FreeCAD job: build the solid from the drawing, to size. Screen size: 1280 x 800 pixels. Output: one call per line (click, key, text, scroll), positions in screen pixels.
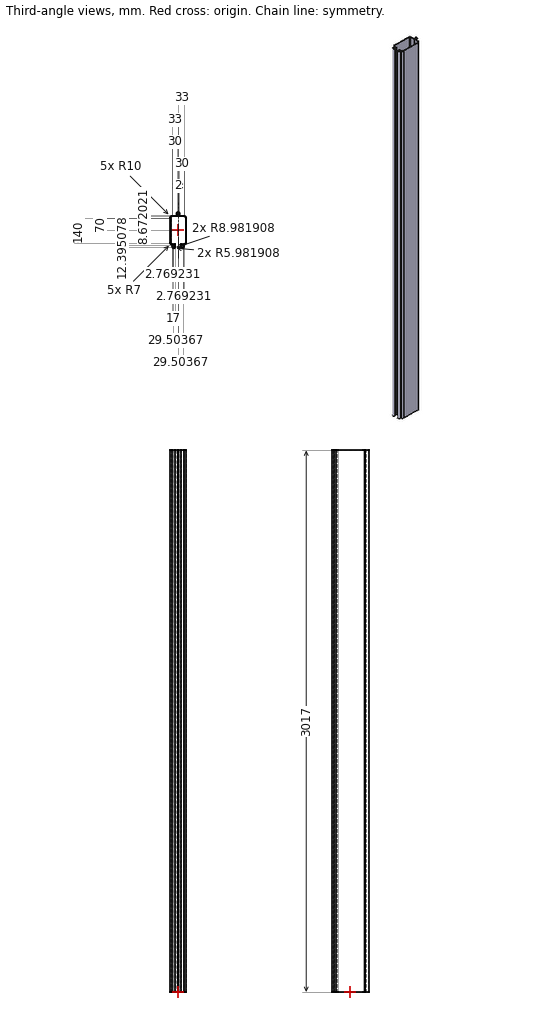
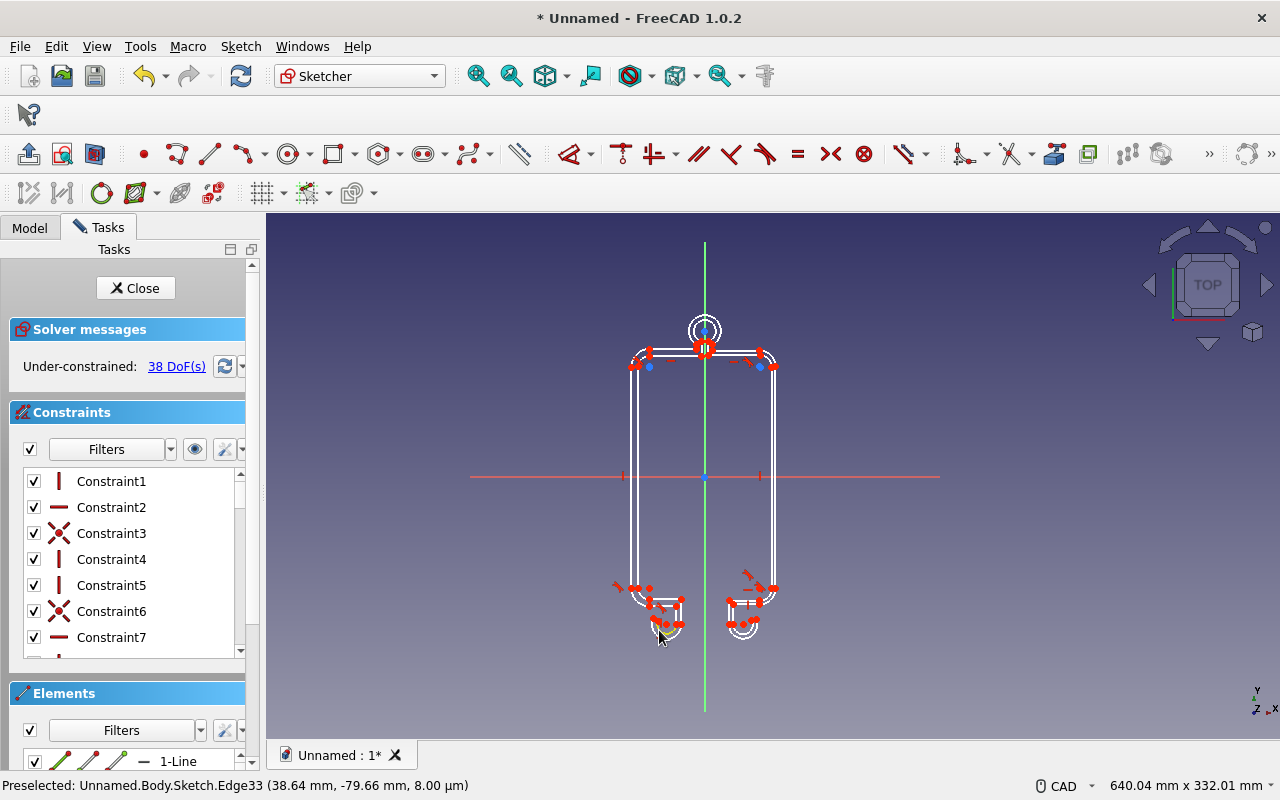
scroll(771, 362, up, 7)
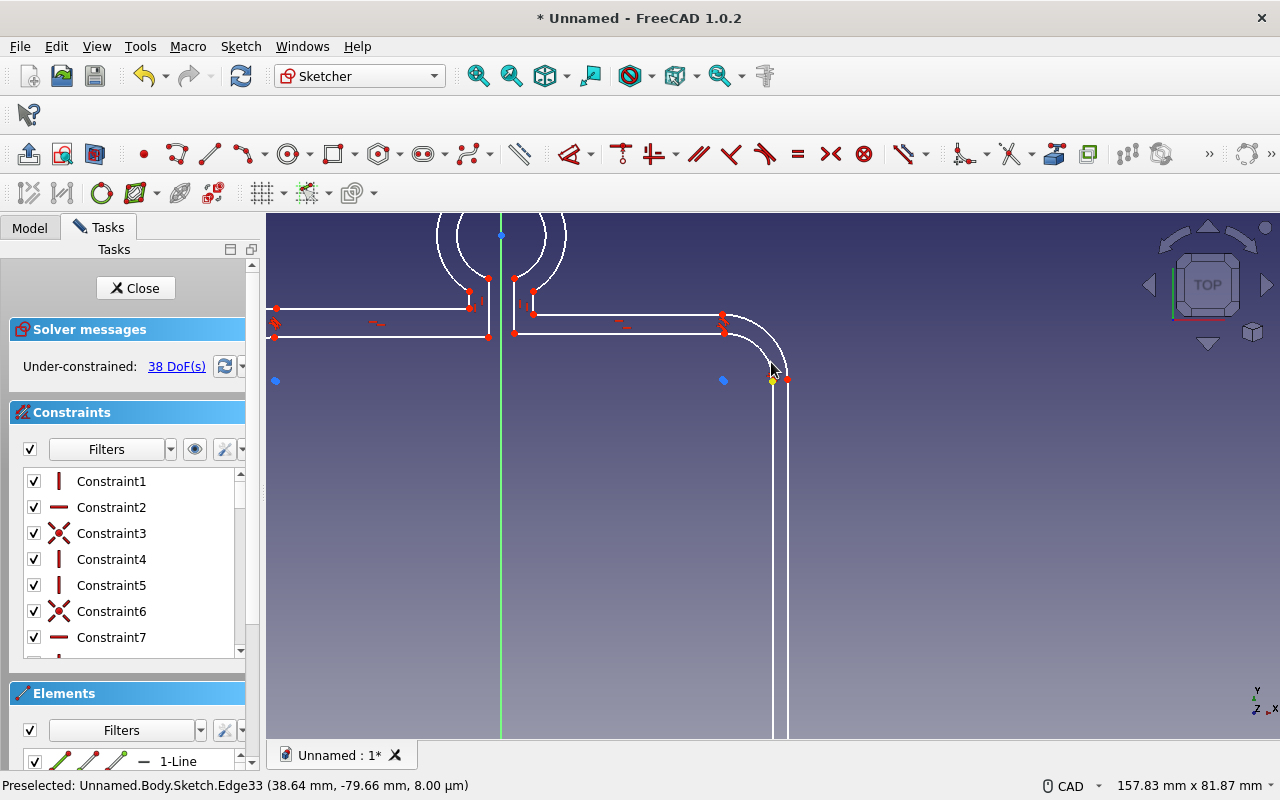
click(768, 360)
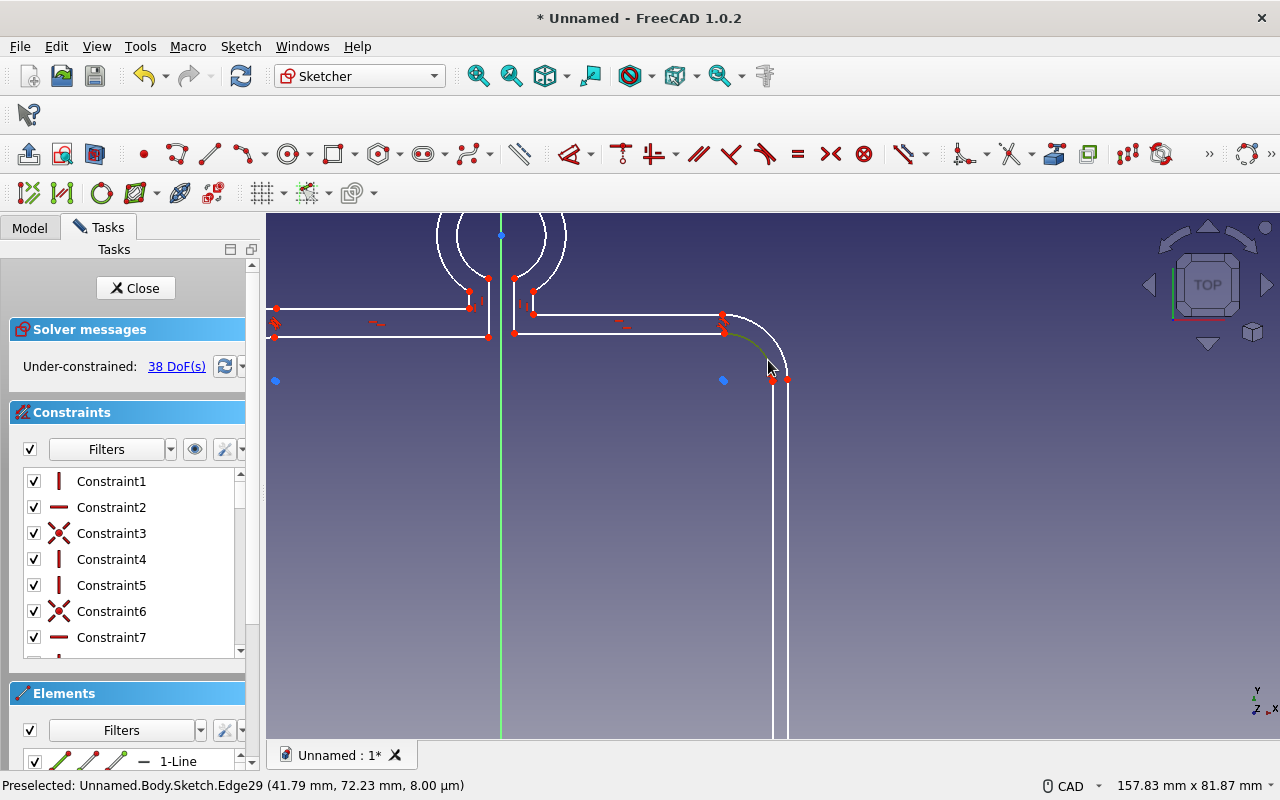
click(780, 350)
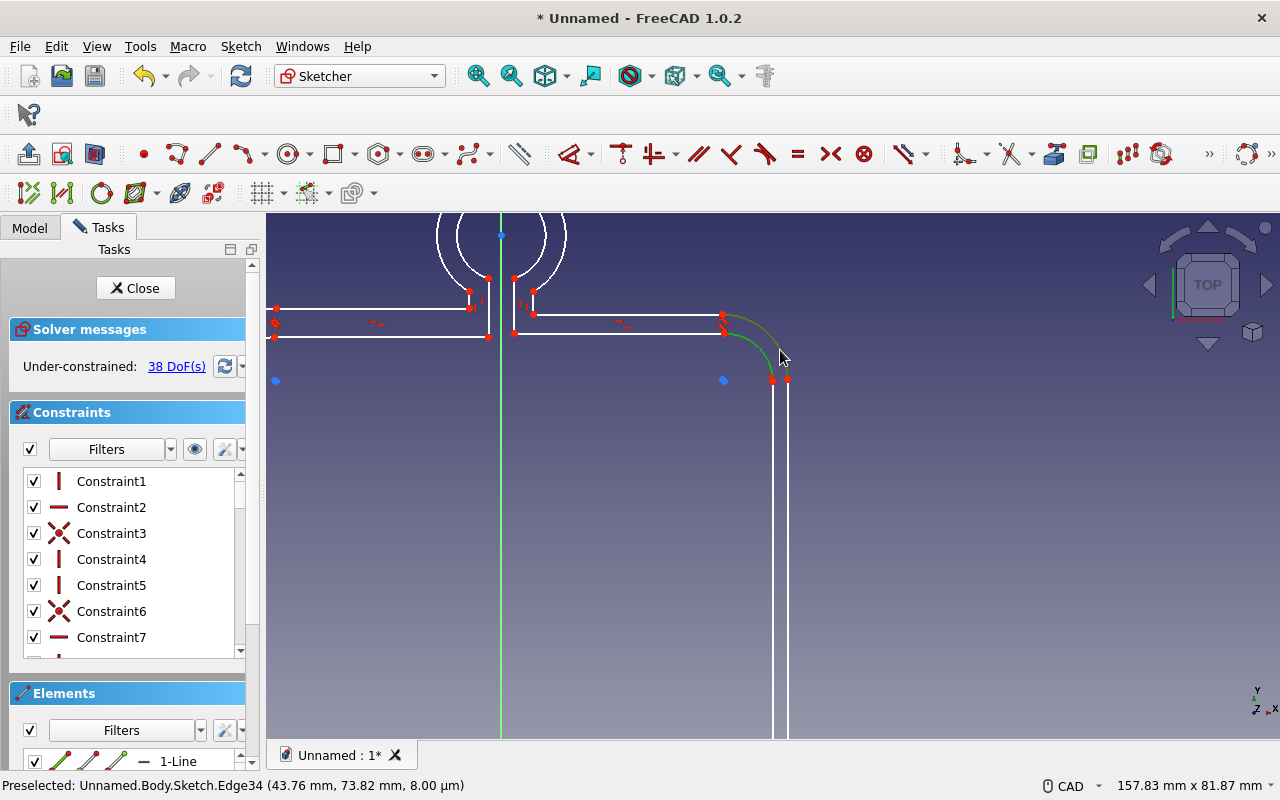
click(621, 154)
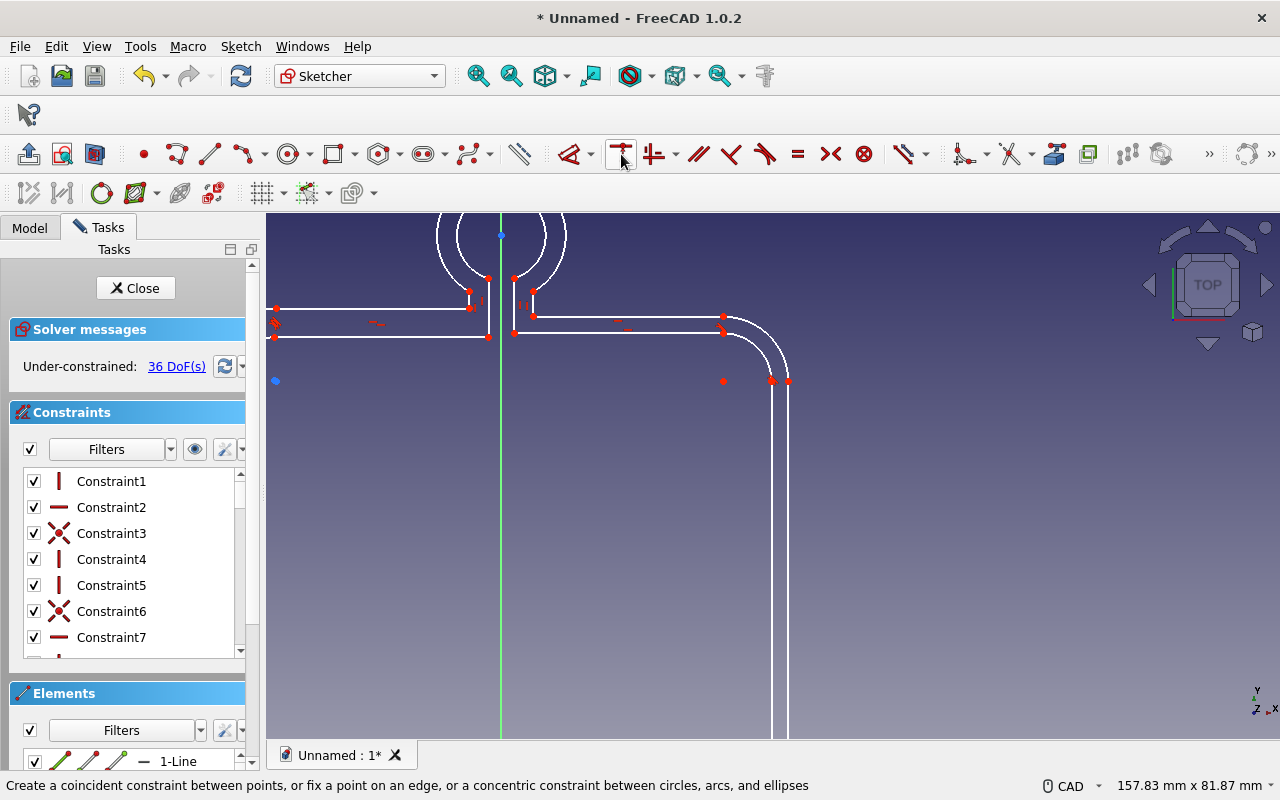
click(545, 242)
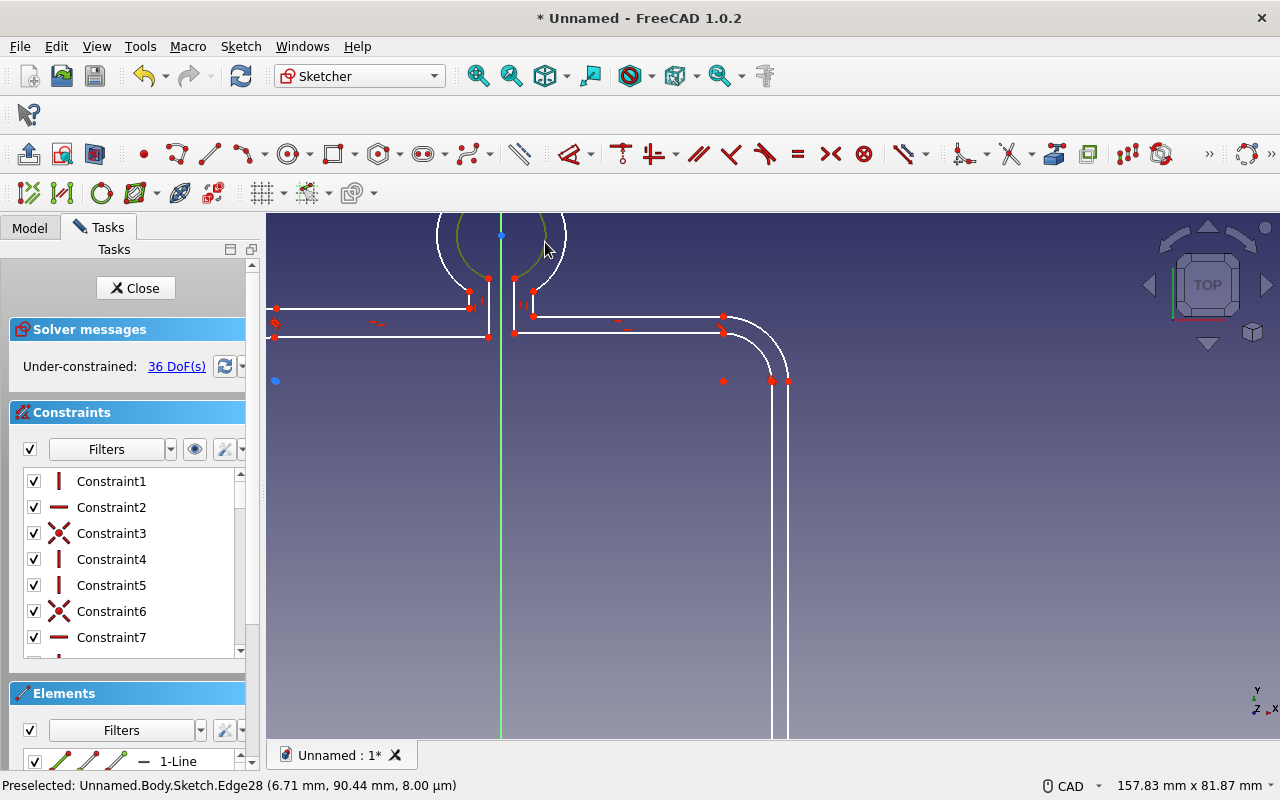
scroll(771, 362, down, 7)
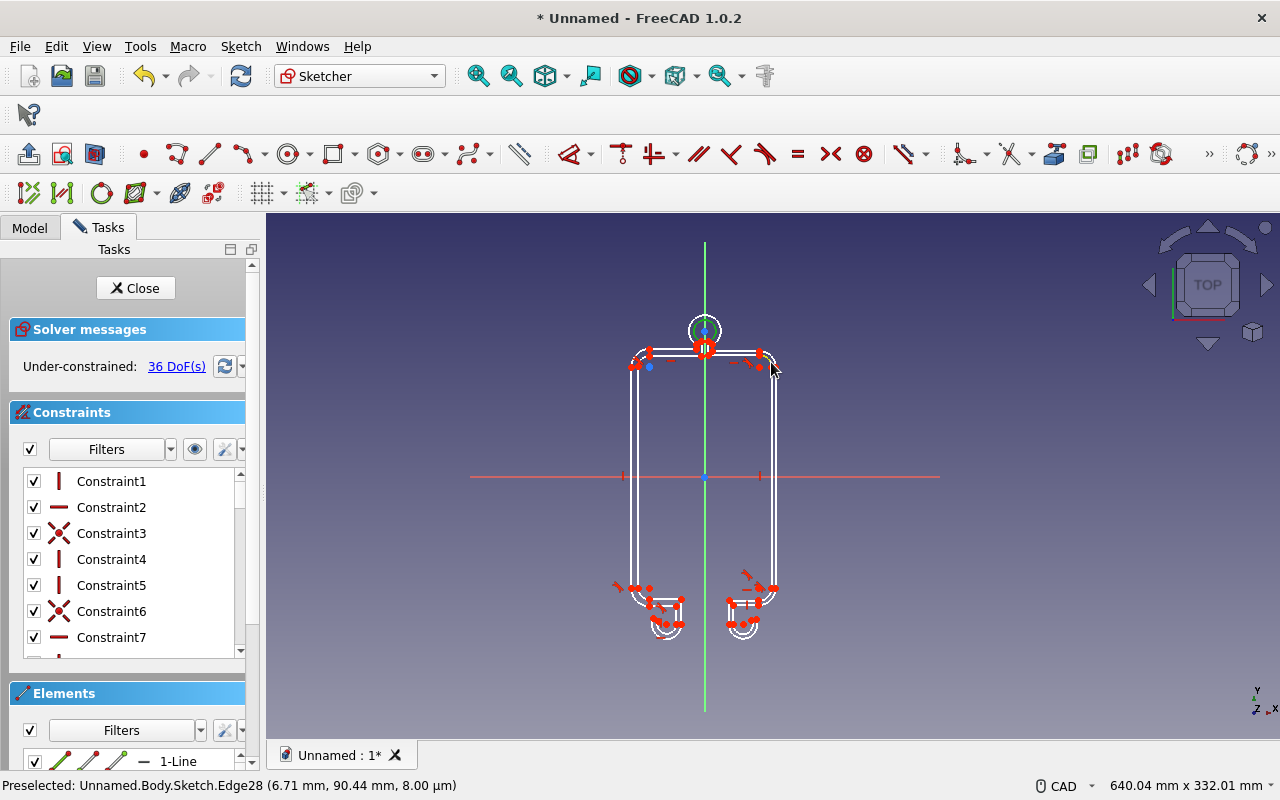
scroll(719, 323, up, 6)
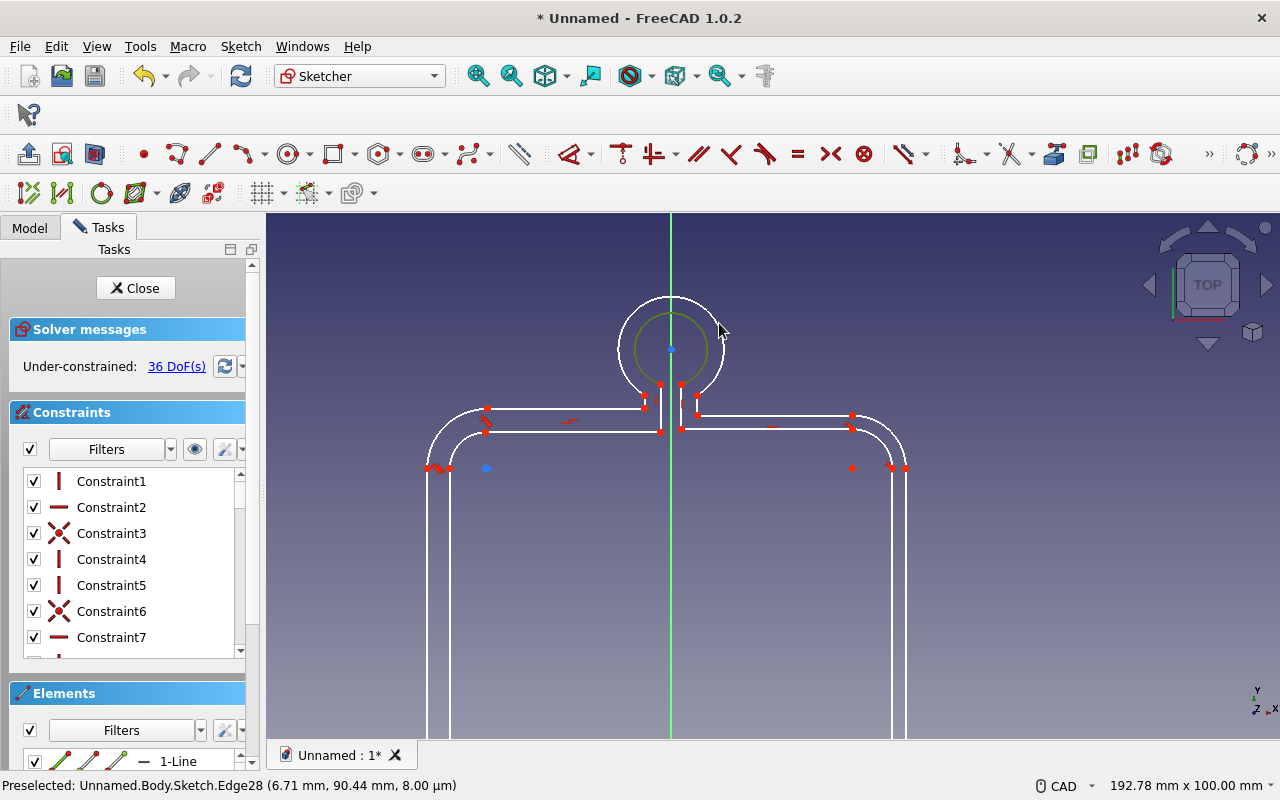
click(717, 323)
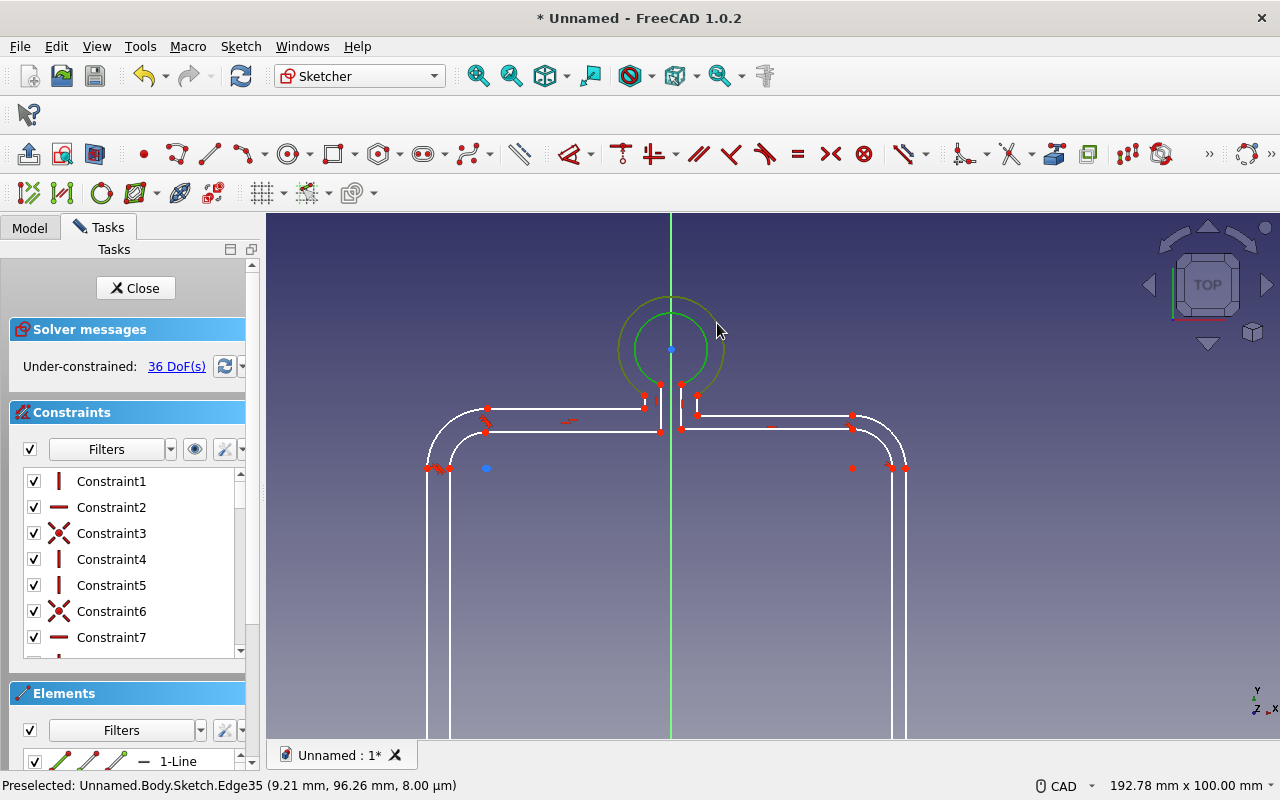
click(621, 154)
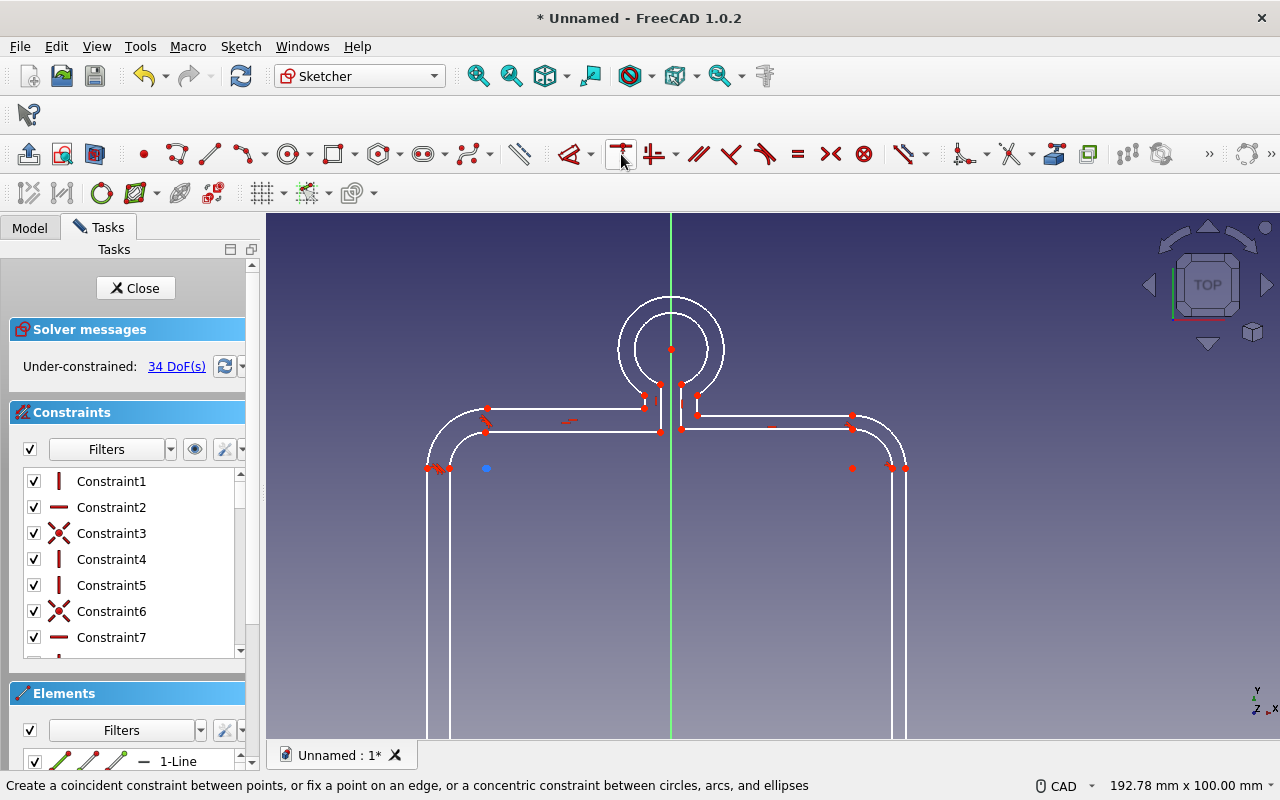
click(469, 436)